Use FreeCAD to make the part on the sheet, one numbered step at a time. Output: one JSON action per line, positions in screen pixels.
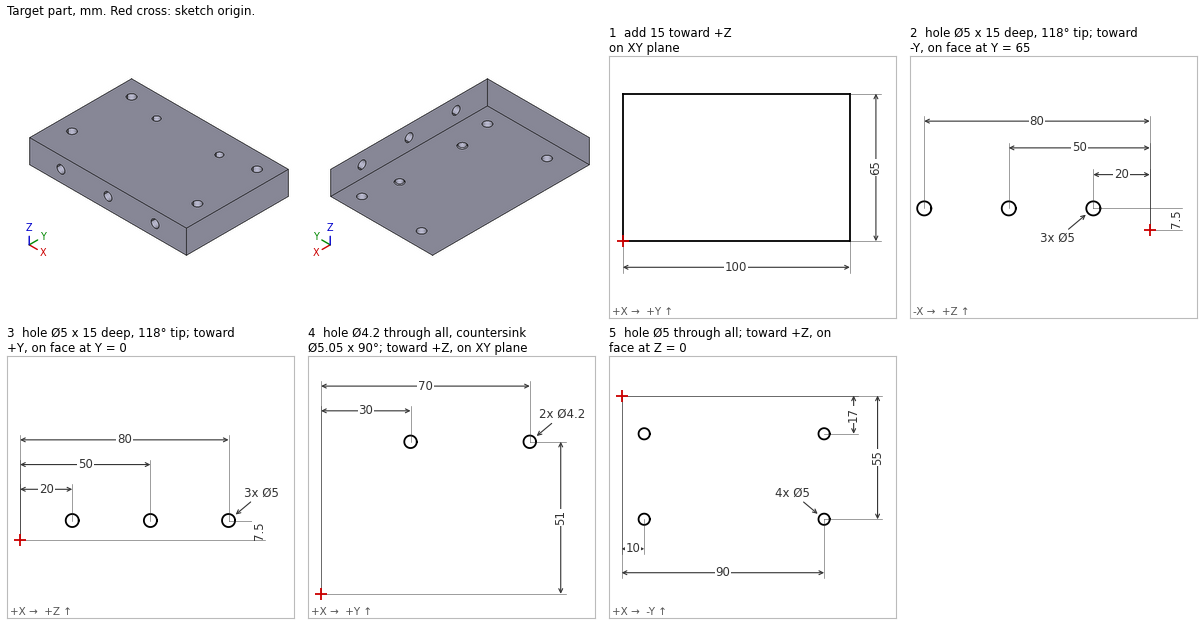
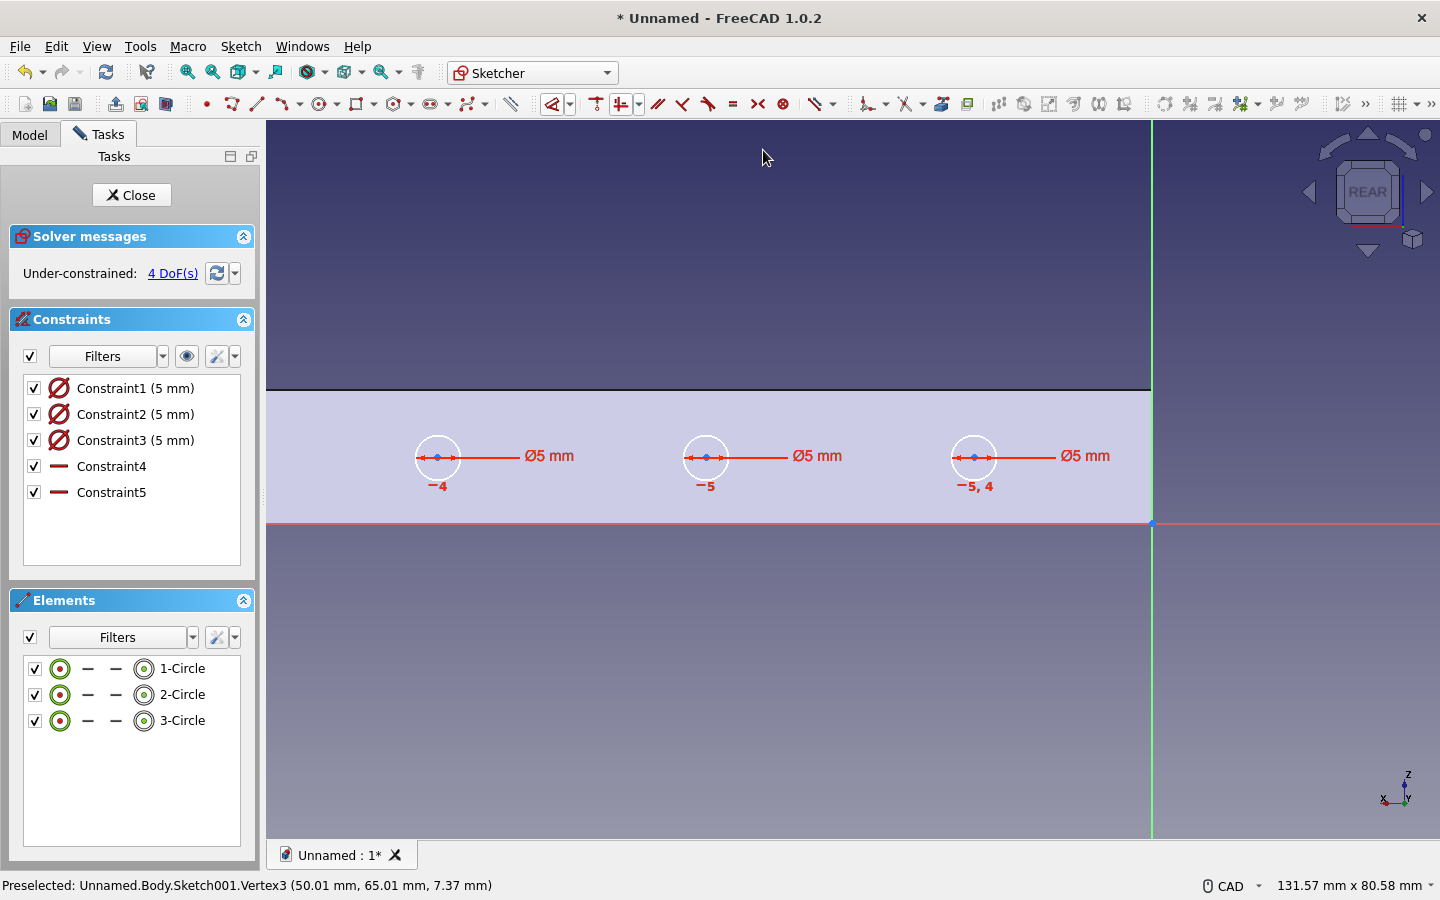
{"action": "left_click", "coordinate": [552, 104]}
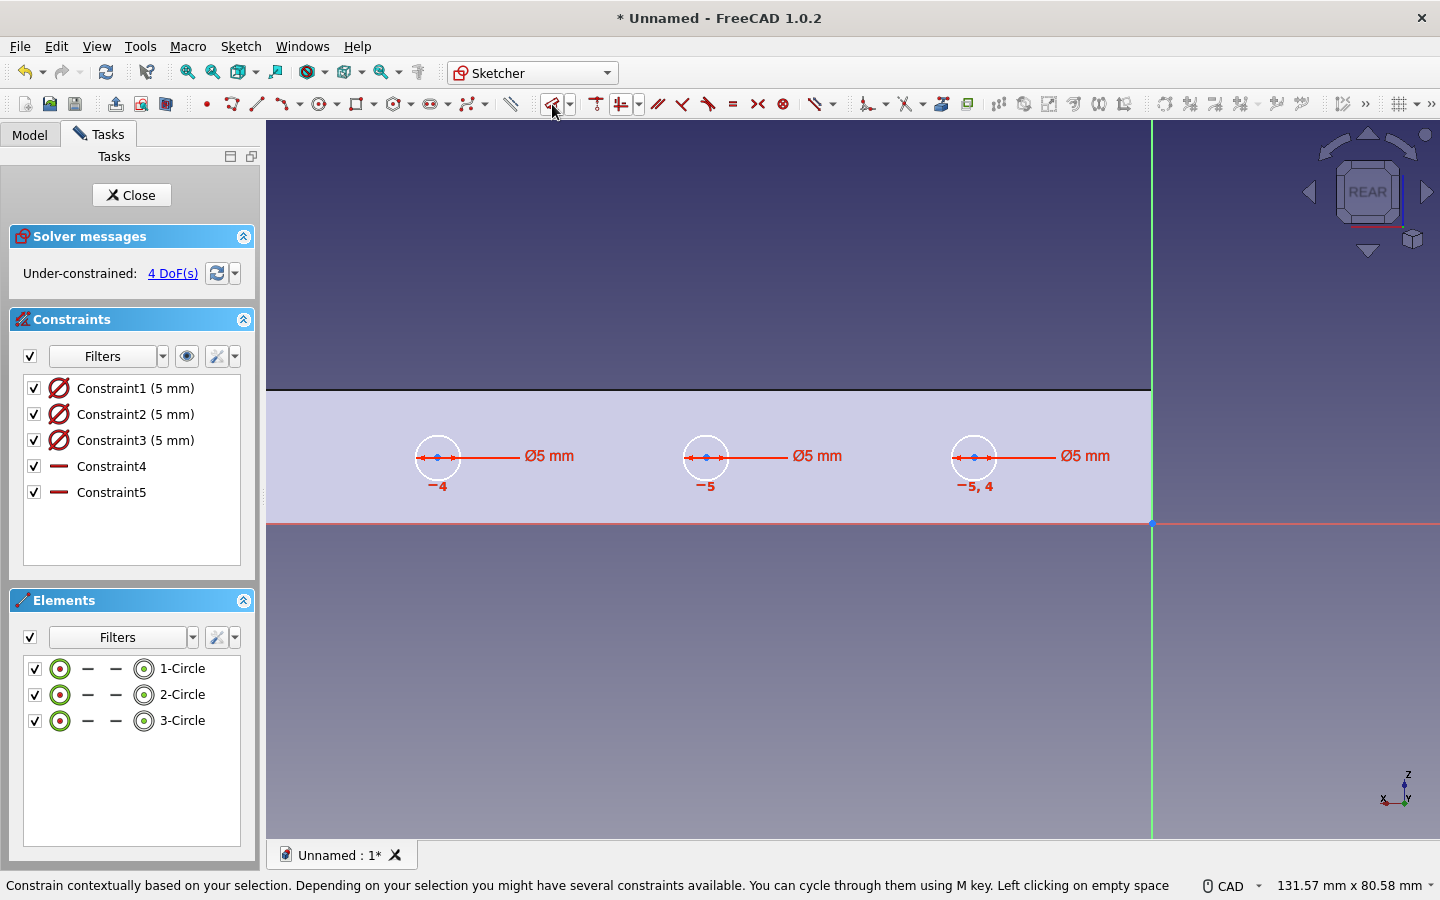
{"action": "left_click", "coordinate": [974, 458]}
{"action": "left_click", "coordinate": [1063, 558]}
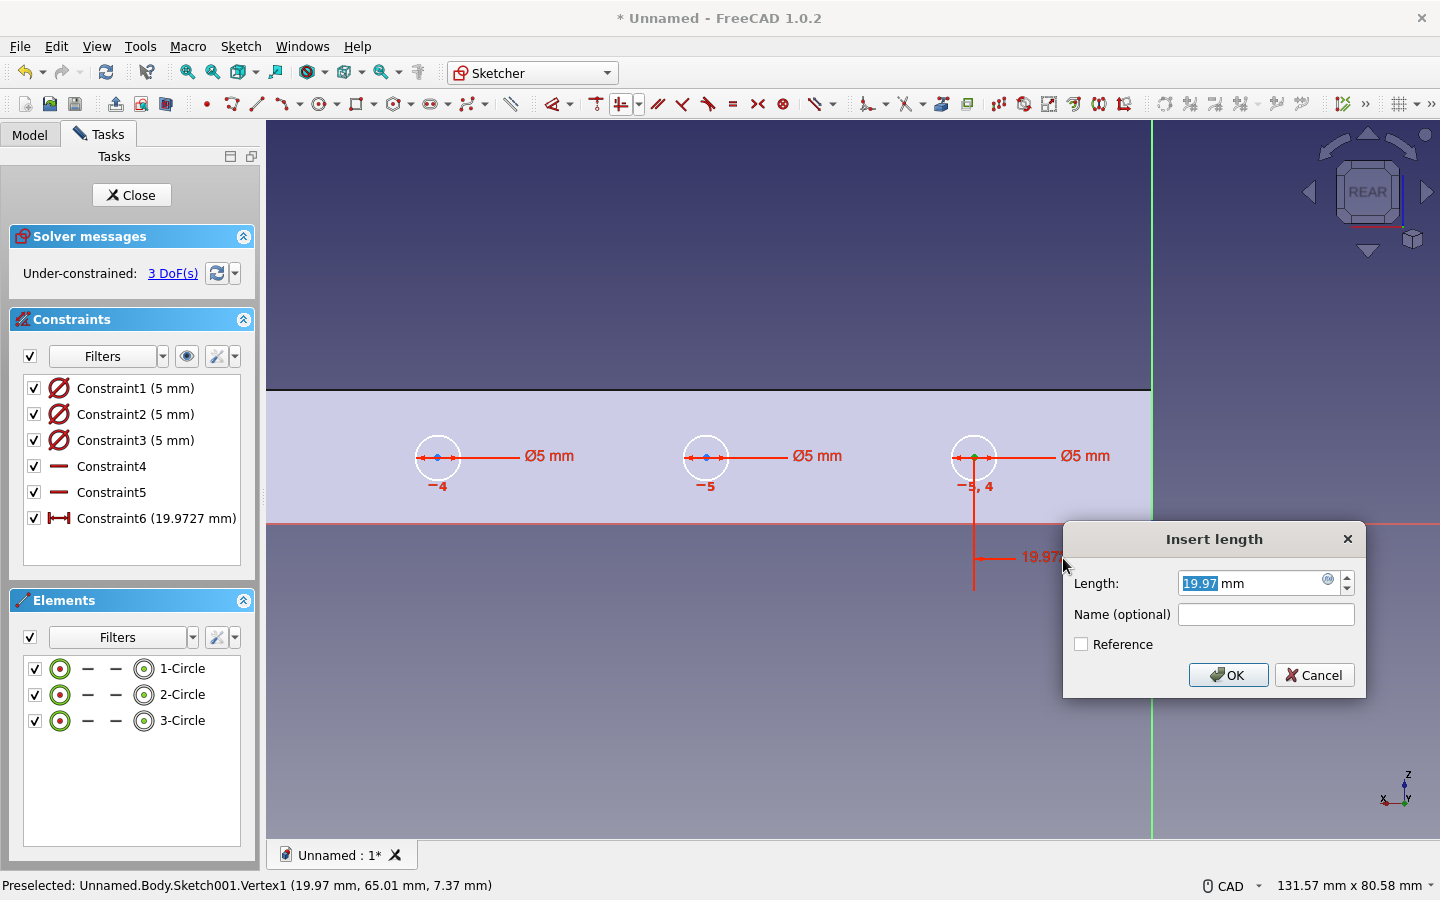
{"action": "type", "text": "20"}
{"action": "key", "text": "Return"}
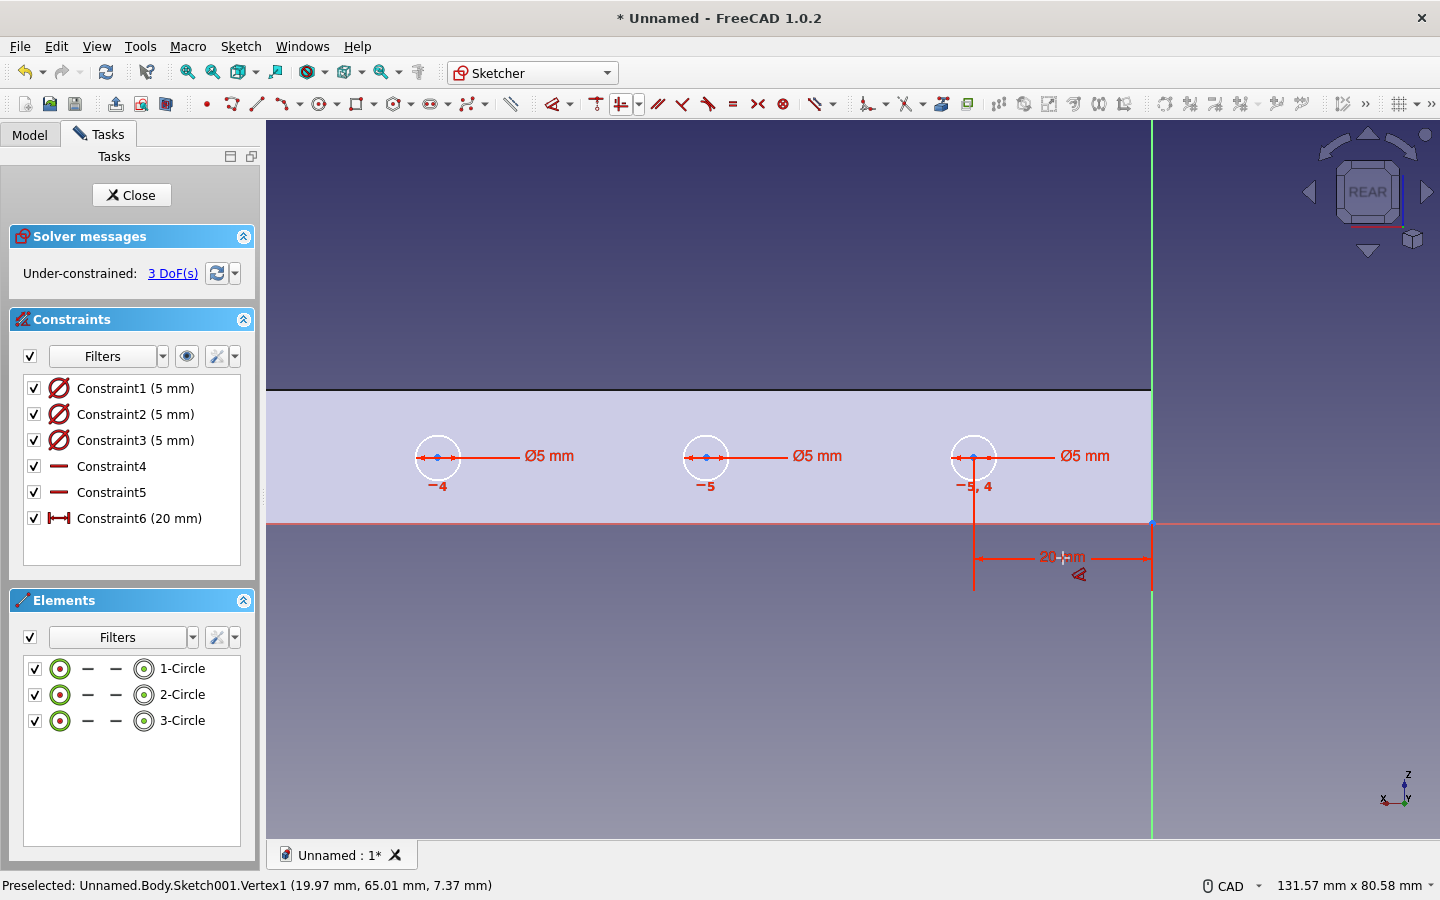
{"action": "left_click", "coordinate": [438, 458]}
{"action": "left_click", "coordinate": [795, 558]}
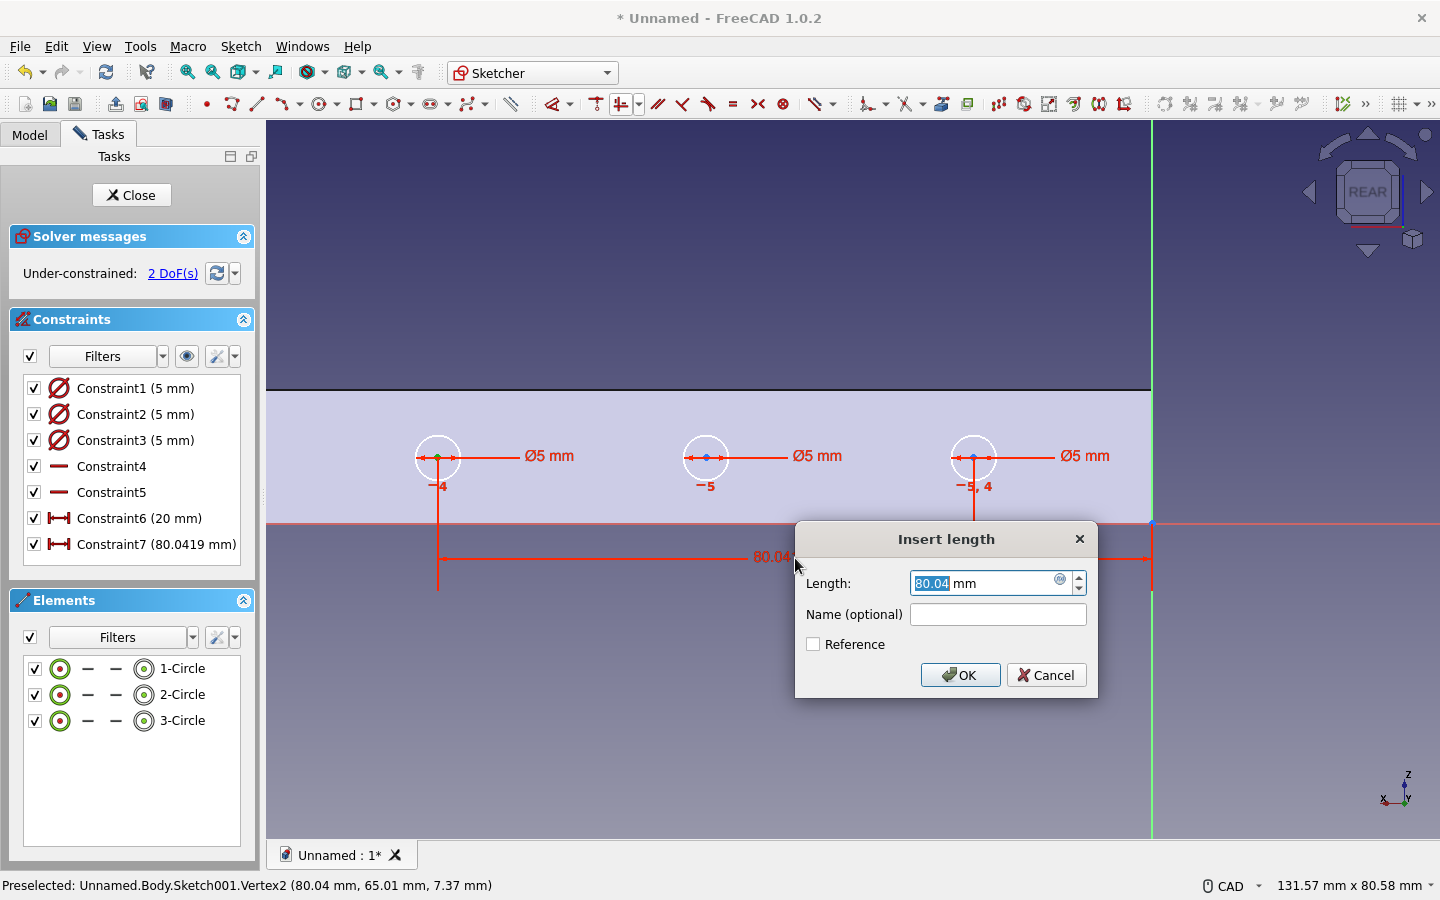
{"action": "type", "text": "80"}
{"action": "key", "text": "Return"}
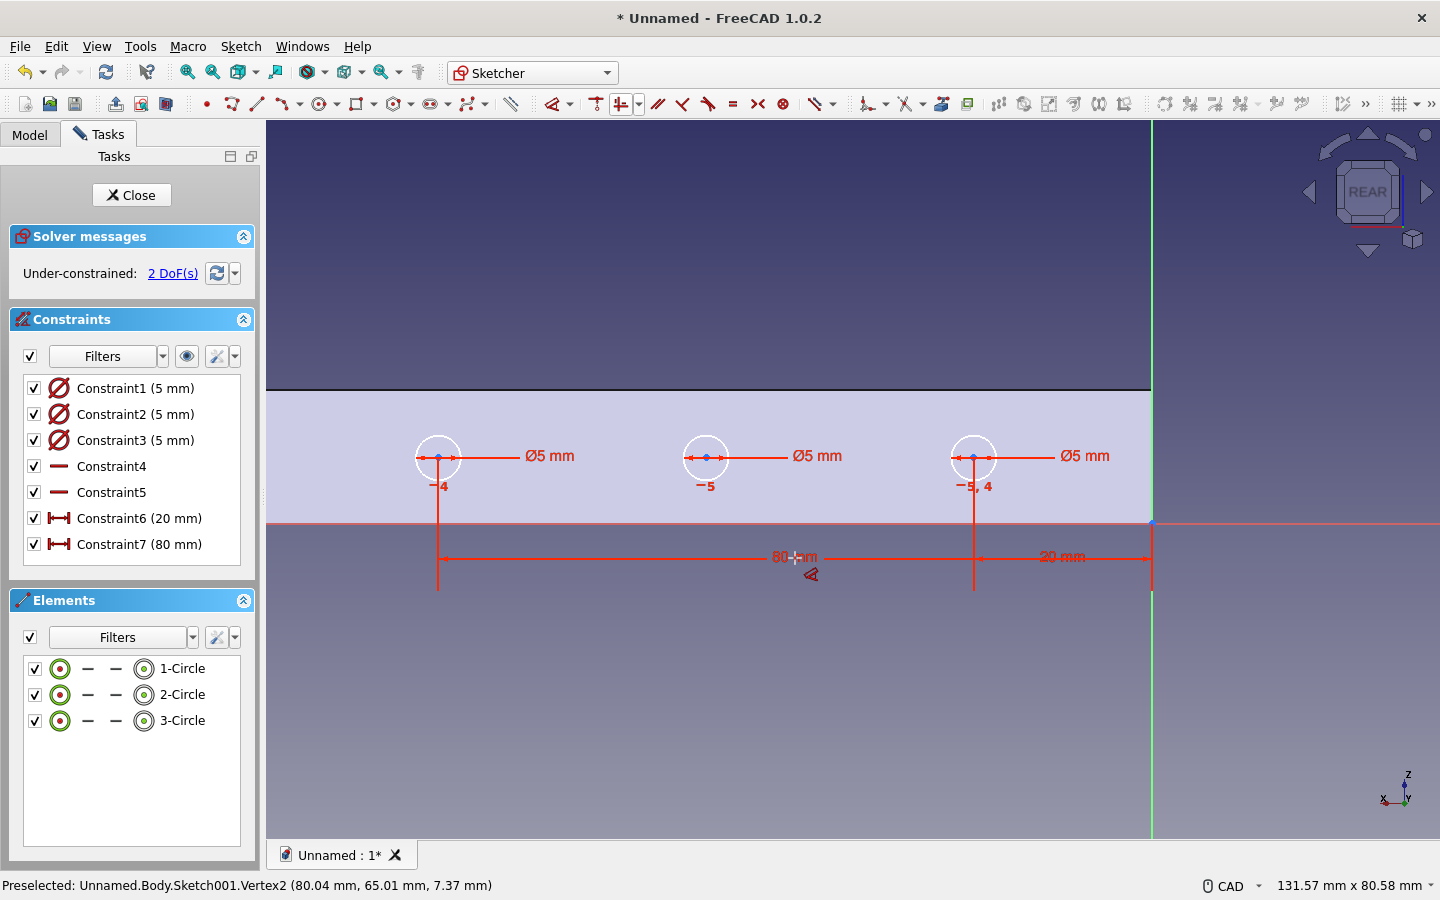
{"action": "left_click", "coordinate": [706, 458]}
{"action": "left_click", "coordinate": [929, 558]}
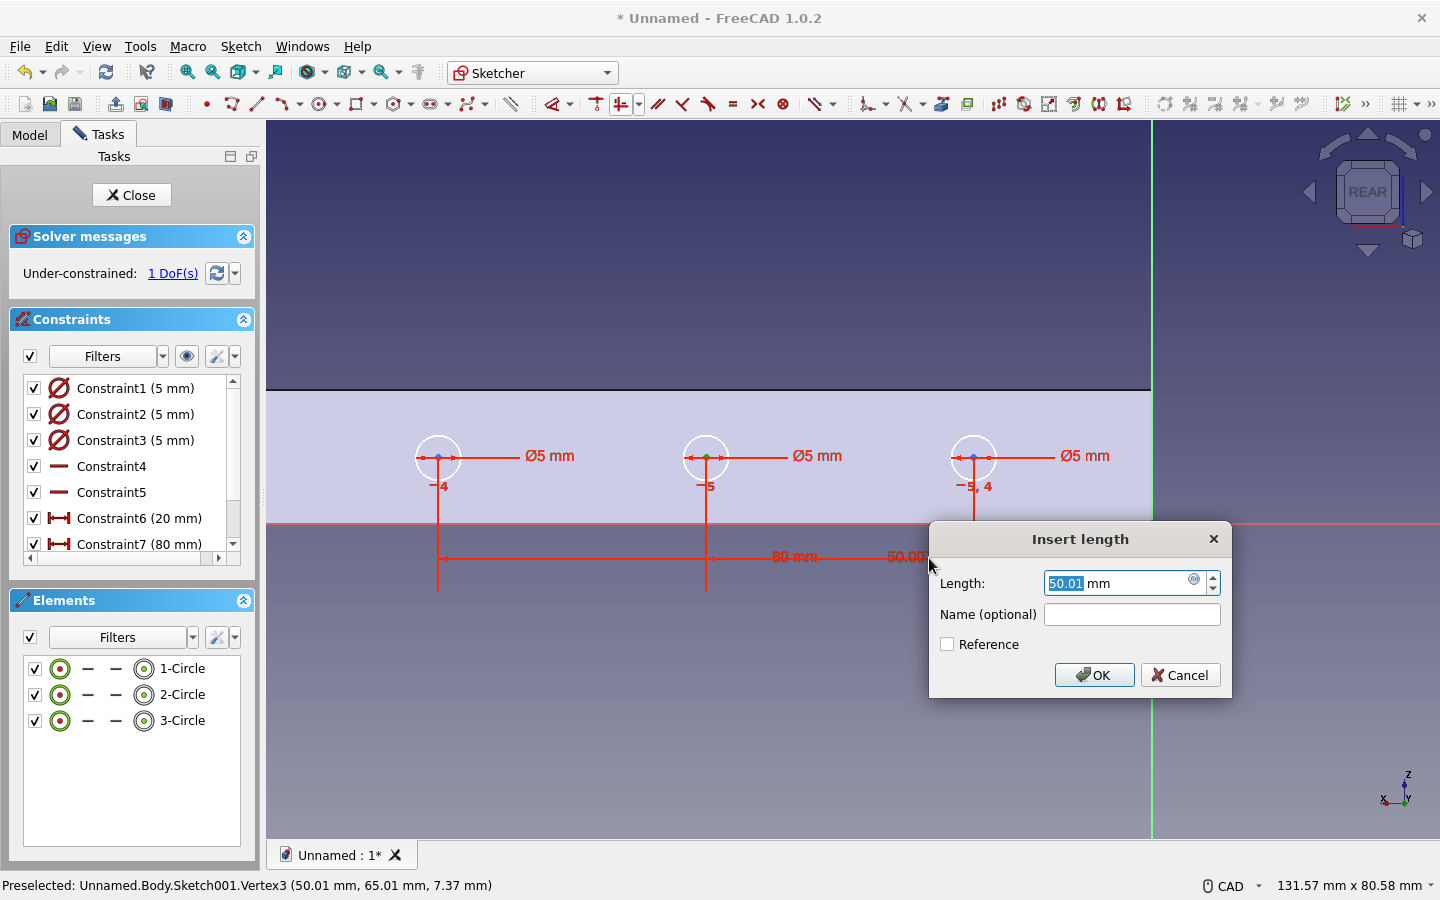
{"action": "type", "text": "50"}
{"action": "key", "text": "Return"}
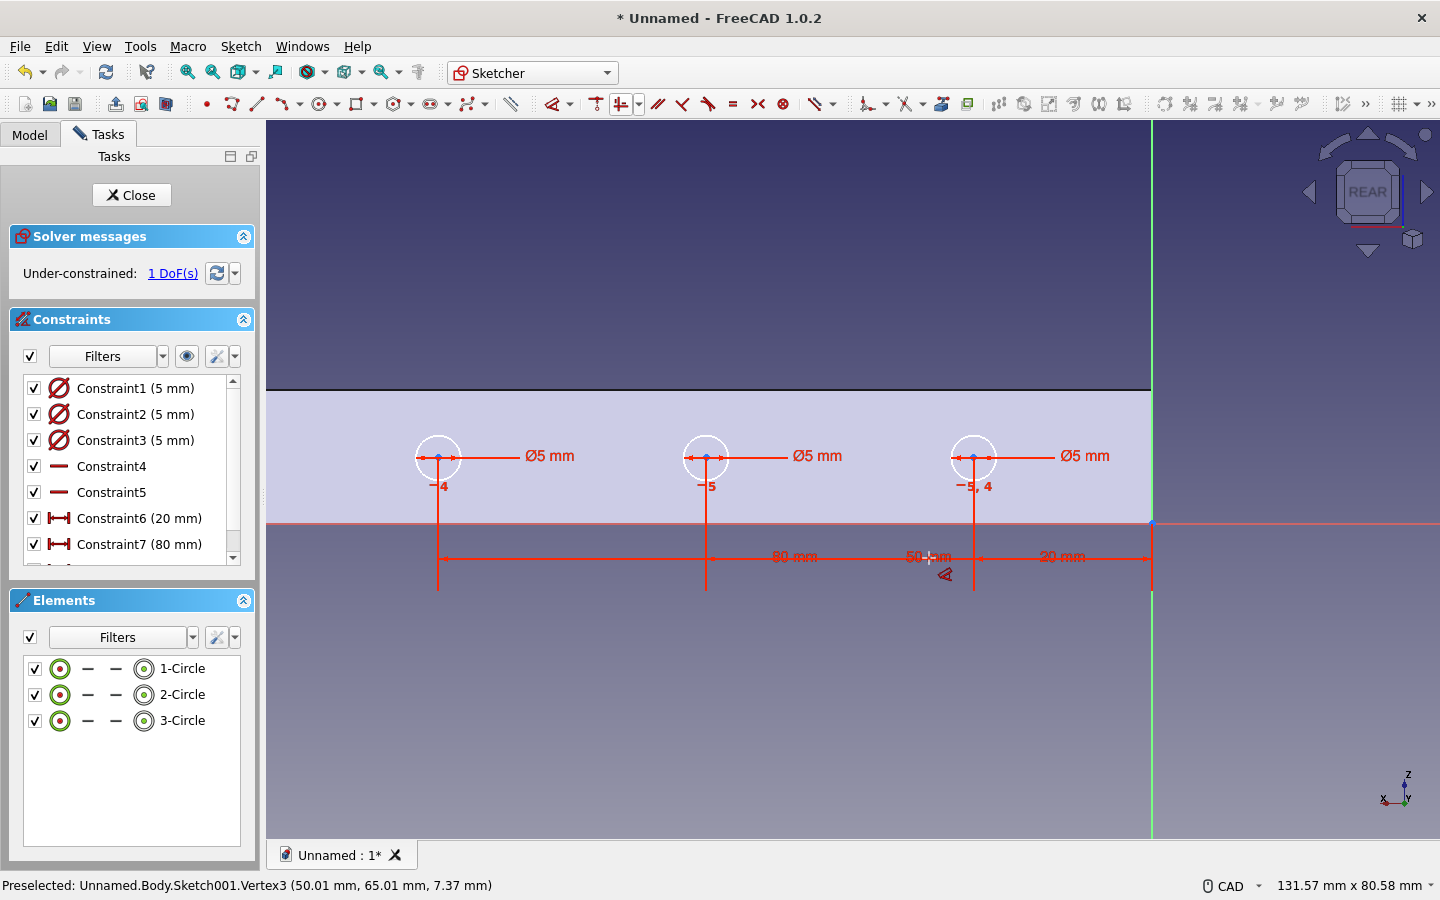
{"action": "left_click", "coordinate": [974, 458]}
{"action": "left_click", "coordinate": [1186, 491]}